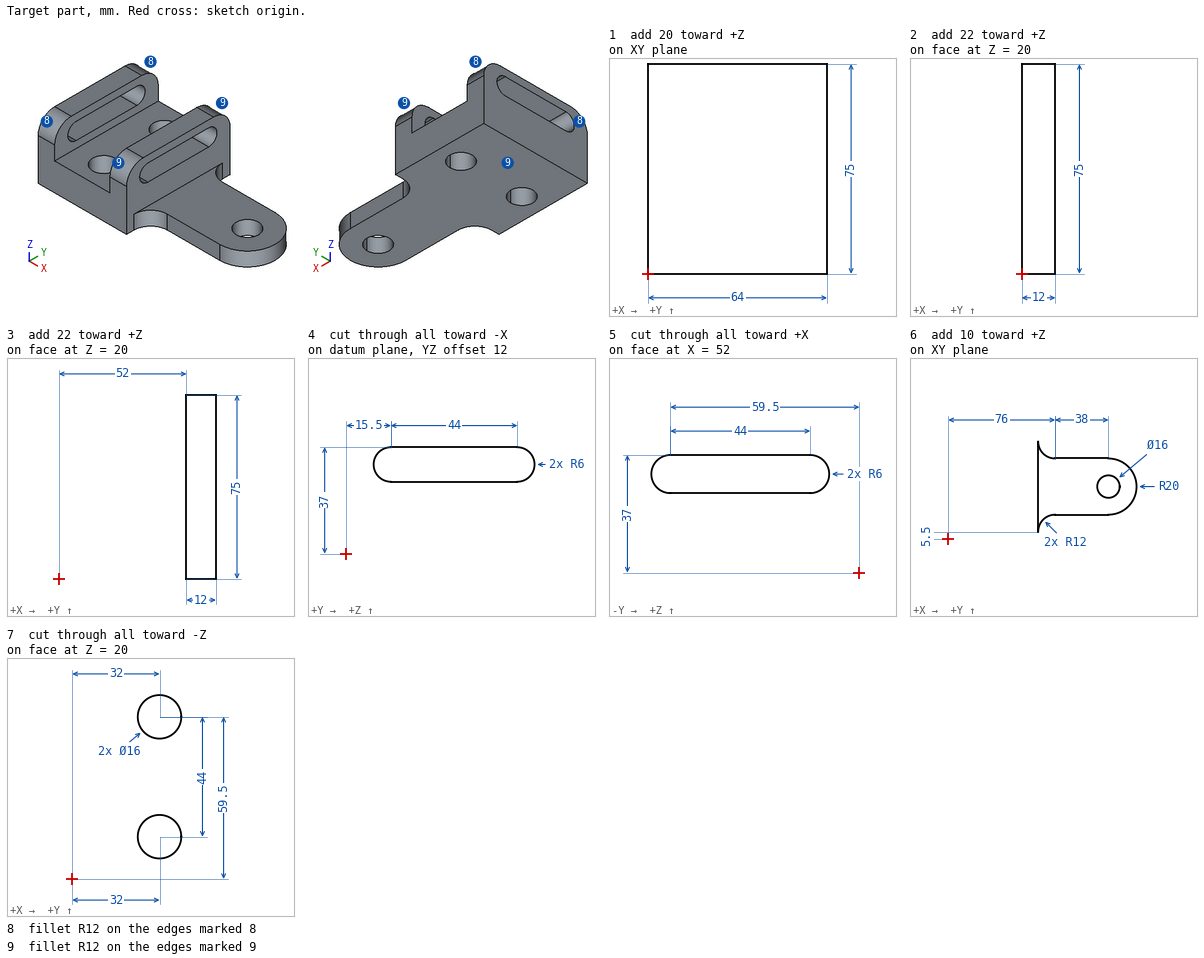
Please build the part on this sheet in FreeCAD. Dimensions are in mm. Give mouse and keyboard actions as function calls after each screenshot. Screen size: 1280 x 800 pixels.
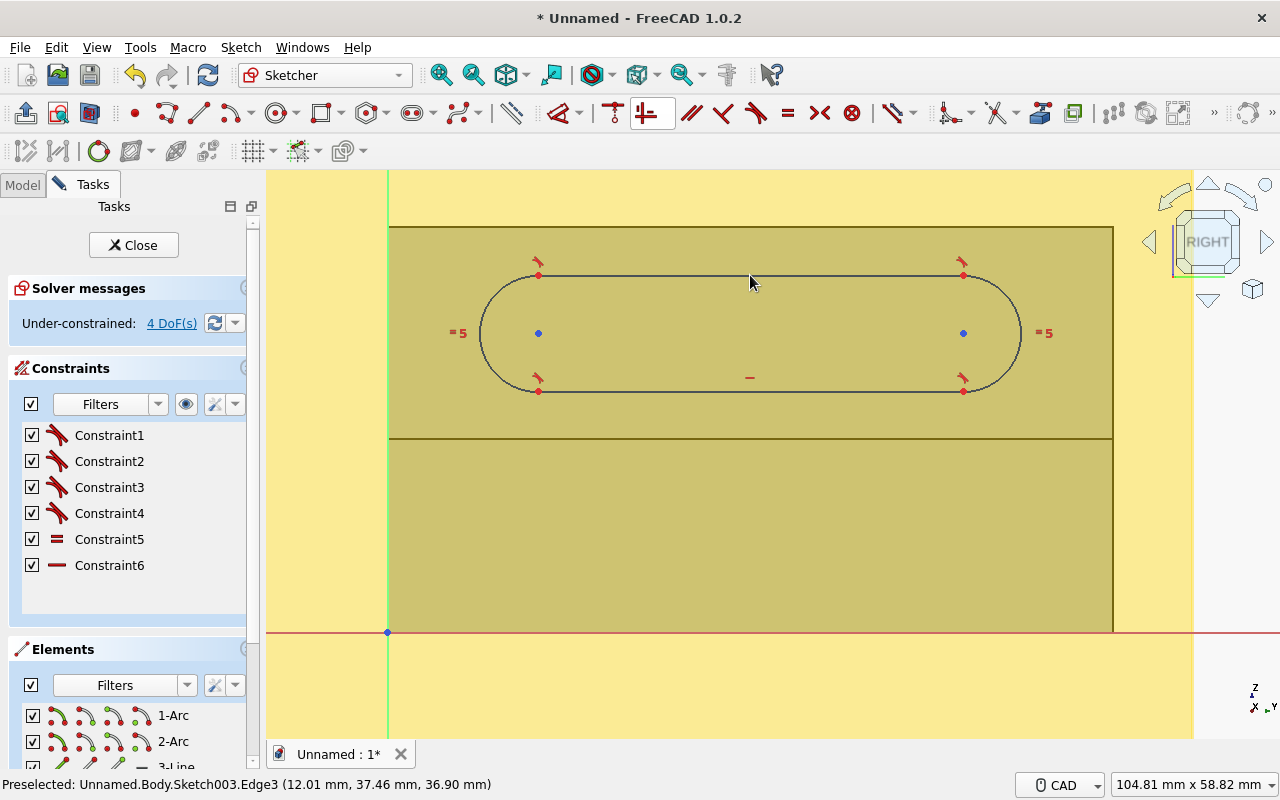
click(558, 114)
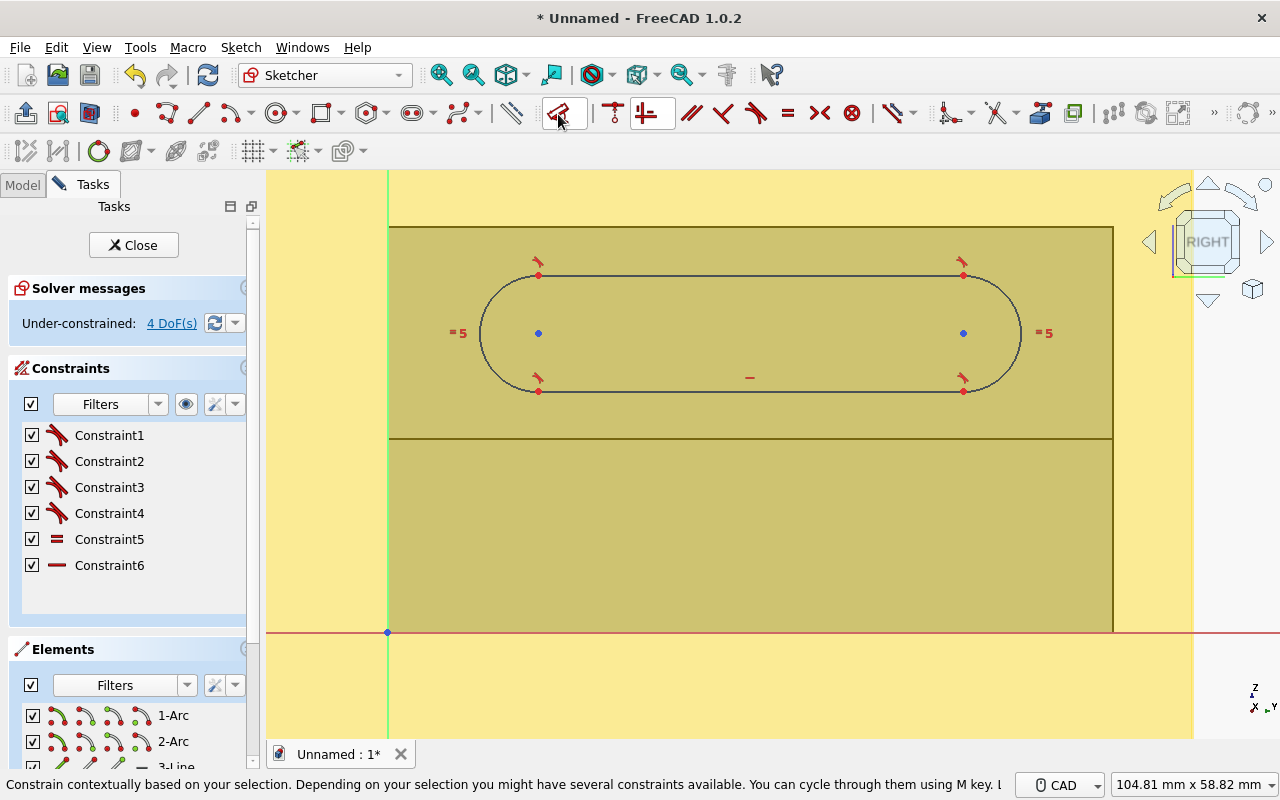
click(491, 300)
click(465, 281)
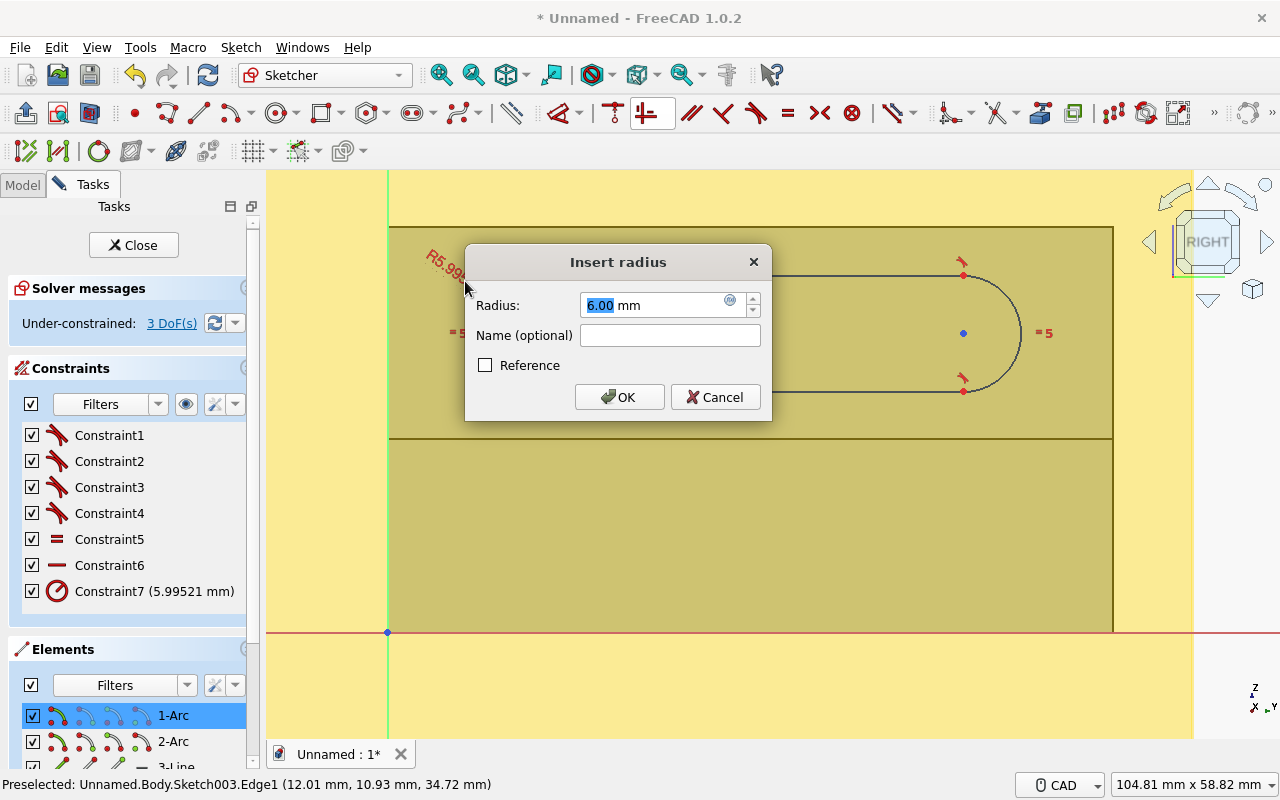
text(6)
key(Return)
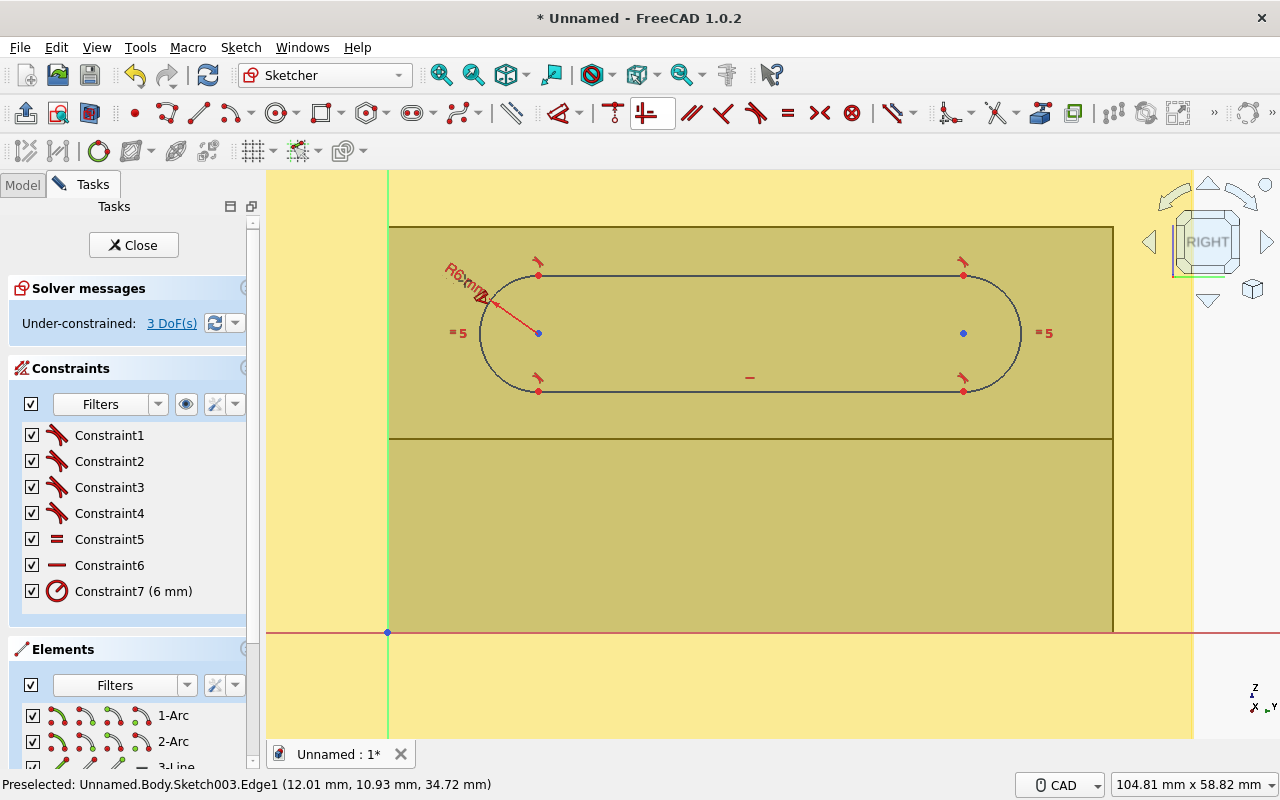
click(665, 276)
click(750, 242)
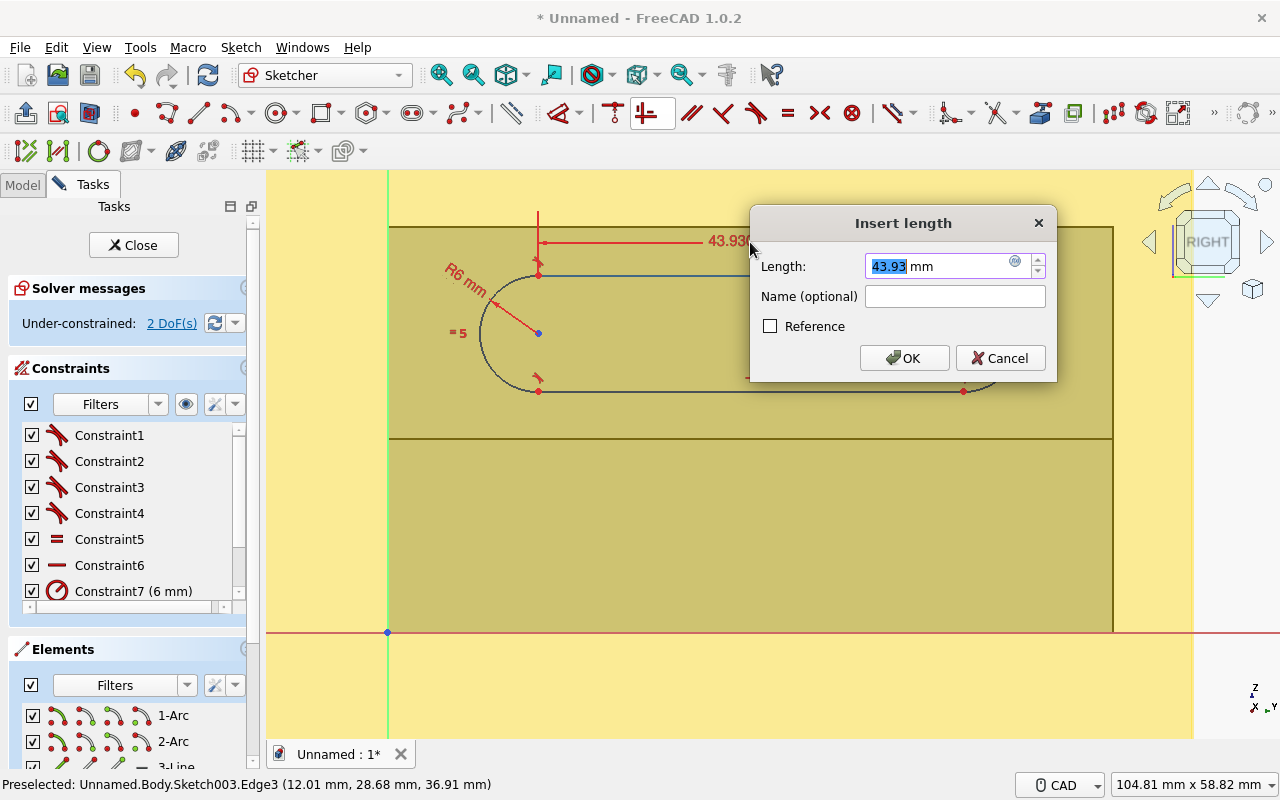
text(44)
key(Return)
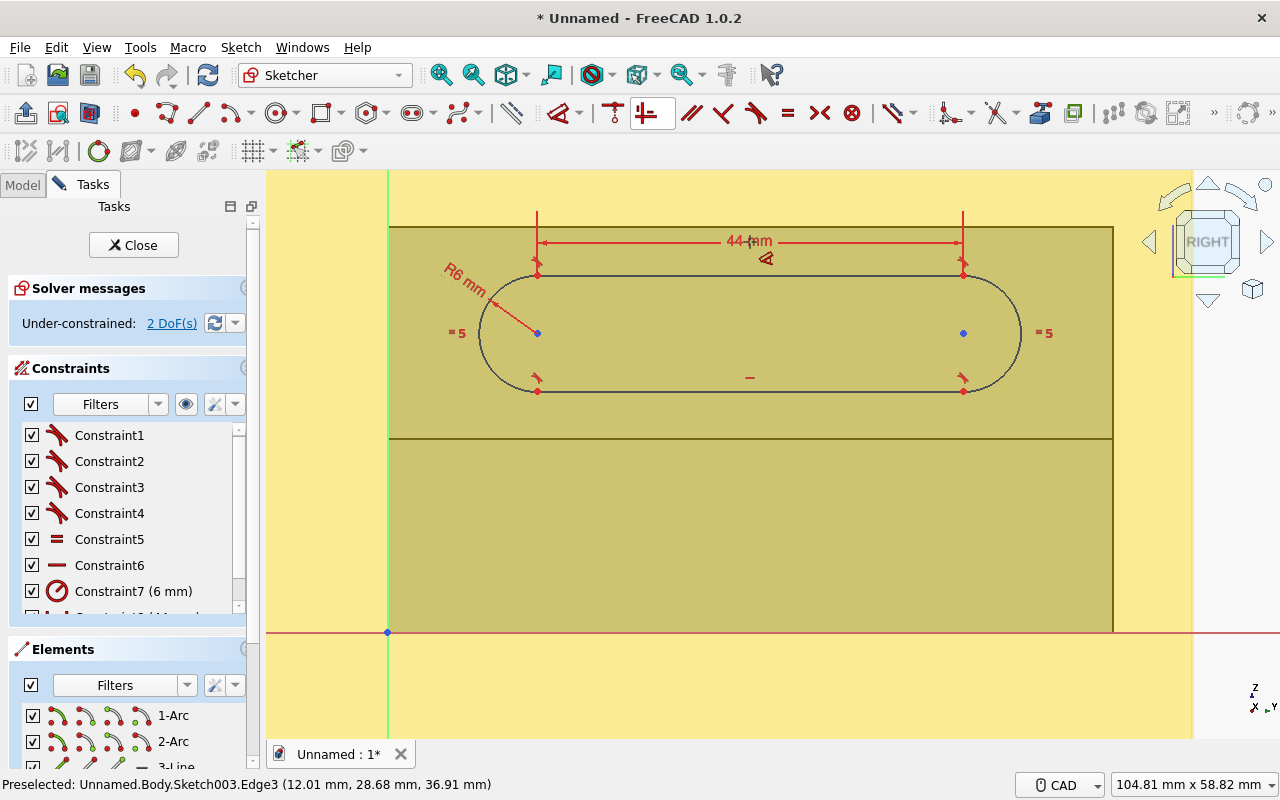
click(537, 276)
click(354, 454)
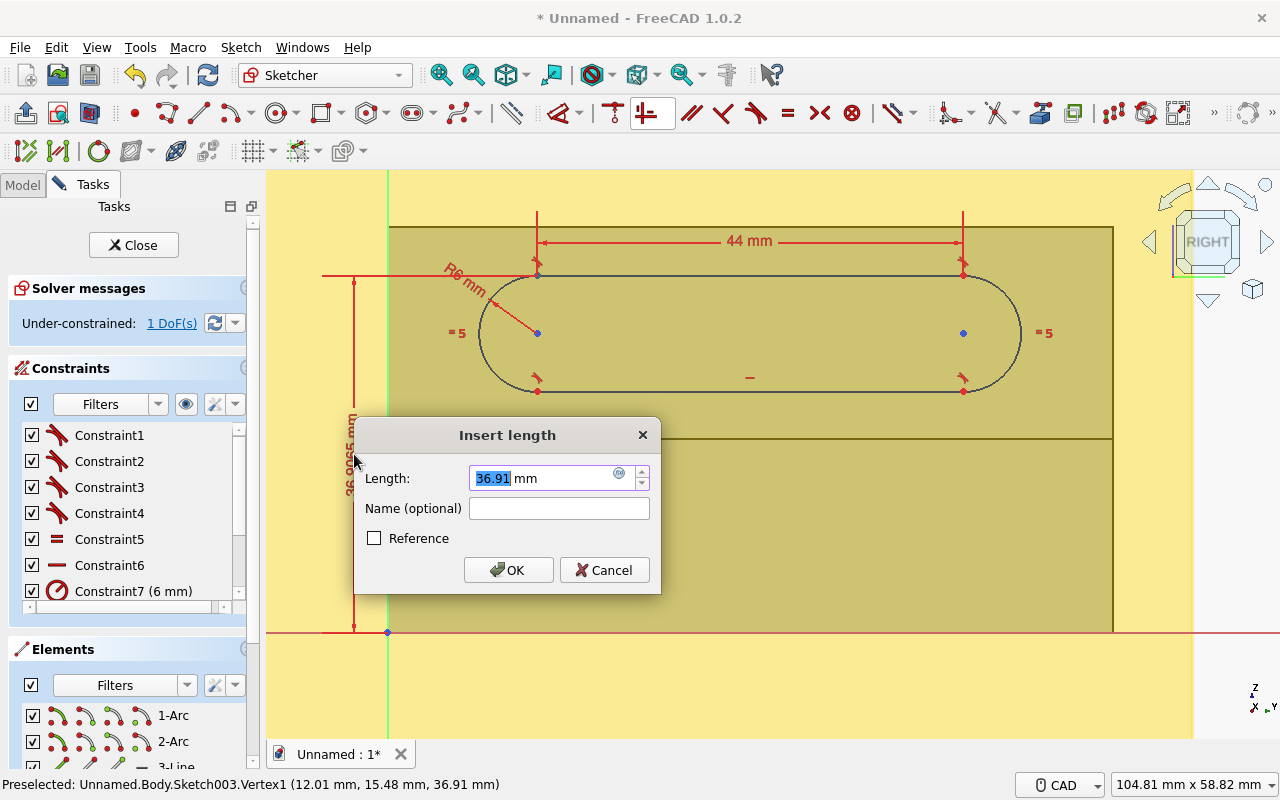
text(37)
key(Return)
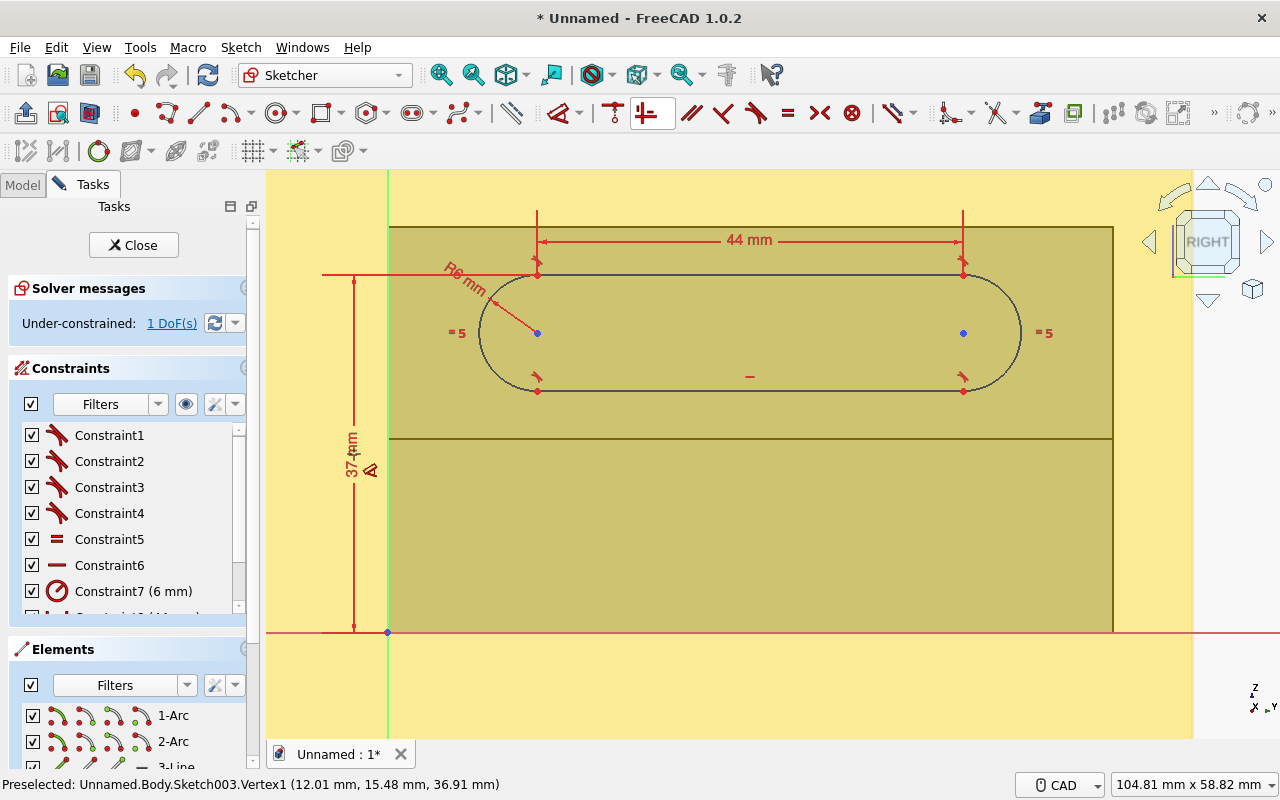
click(537, 275)
click(462, 667)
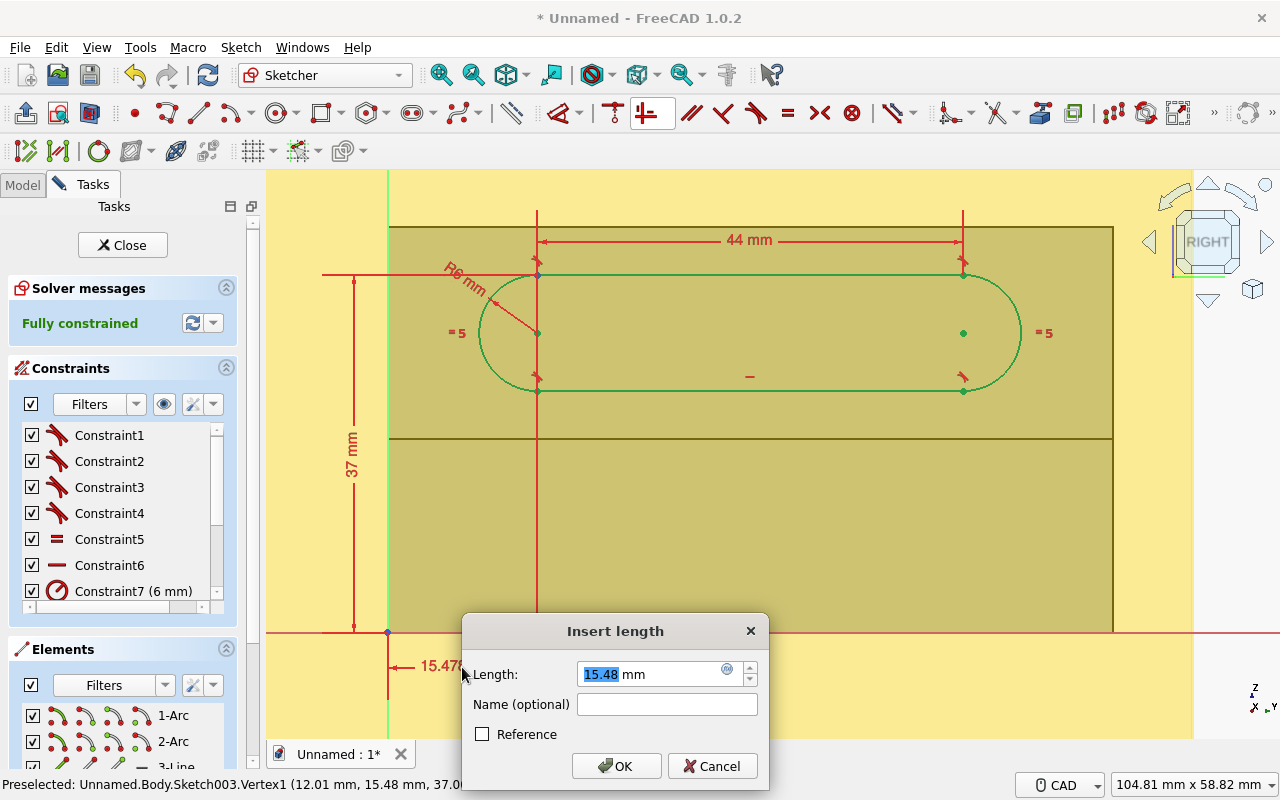
text(15.5)
key(Return)
key(Escape)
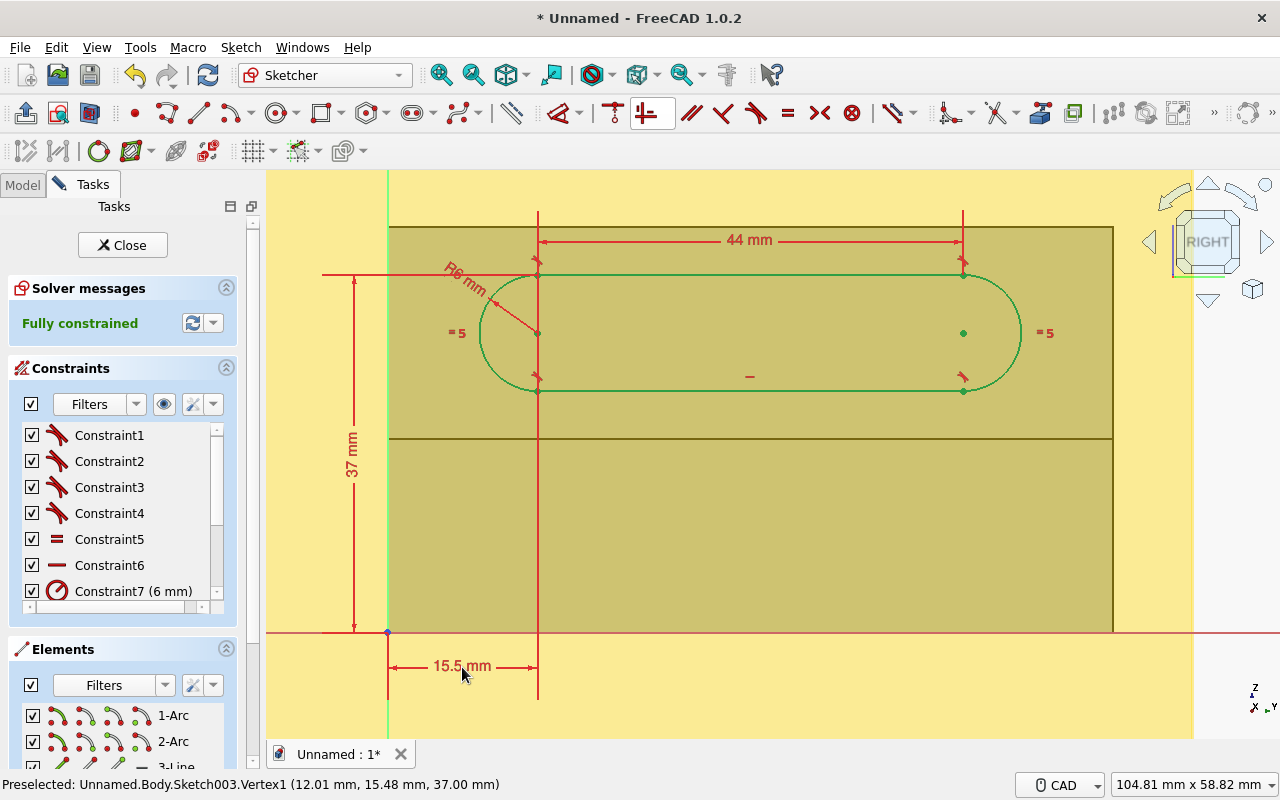
click(123, 245)